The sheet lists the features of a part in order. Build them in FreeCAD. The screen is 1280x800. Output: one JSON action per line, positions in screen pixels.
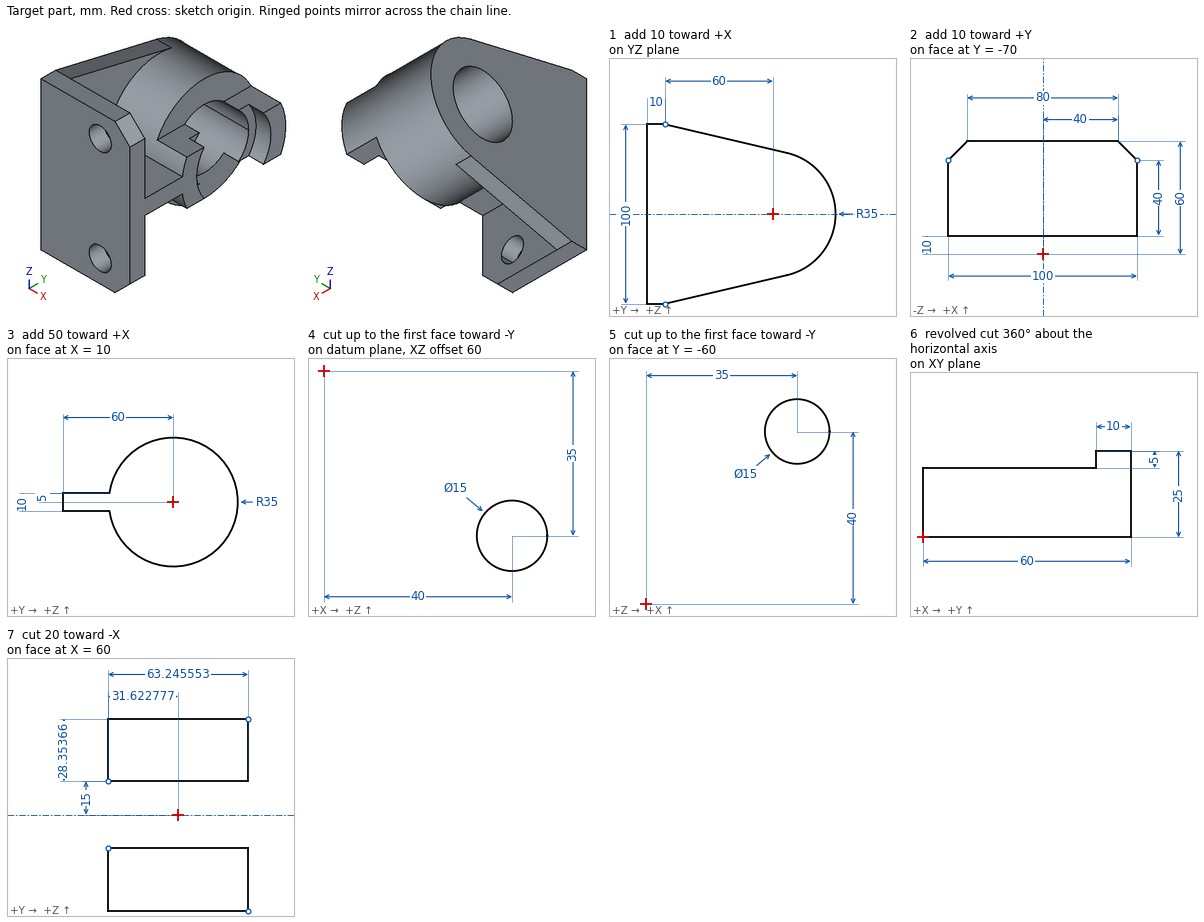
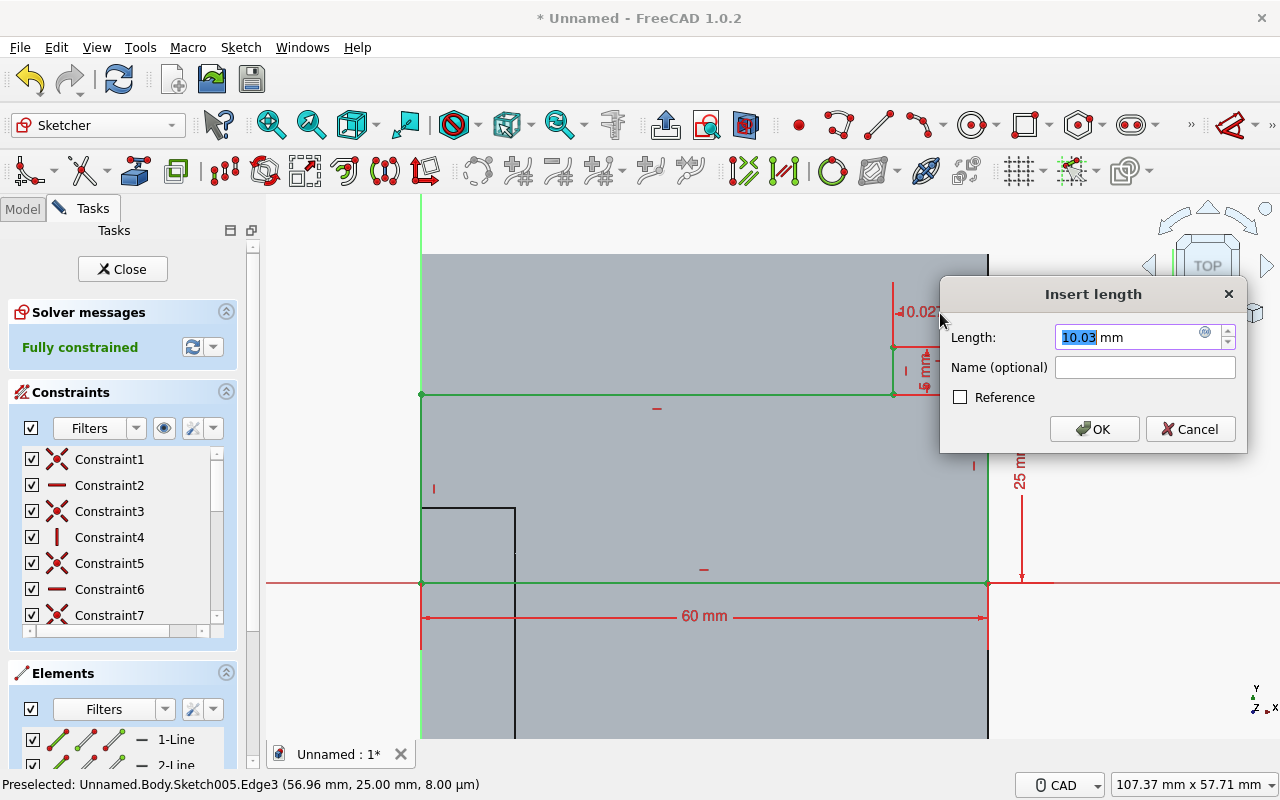
{"action": "type", "text": "10"}
{"action": "key", "text": "Return"}
{"action": "key", "text": "Escape"}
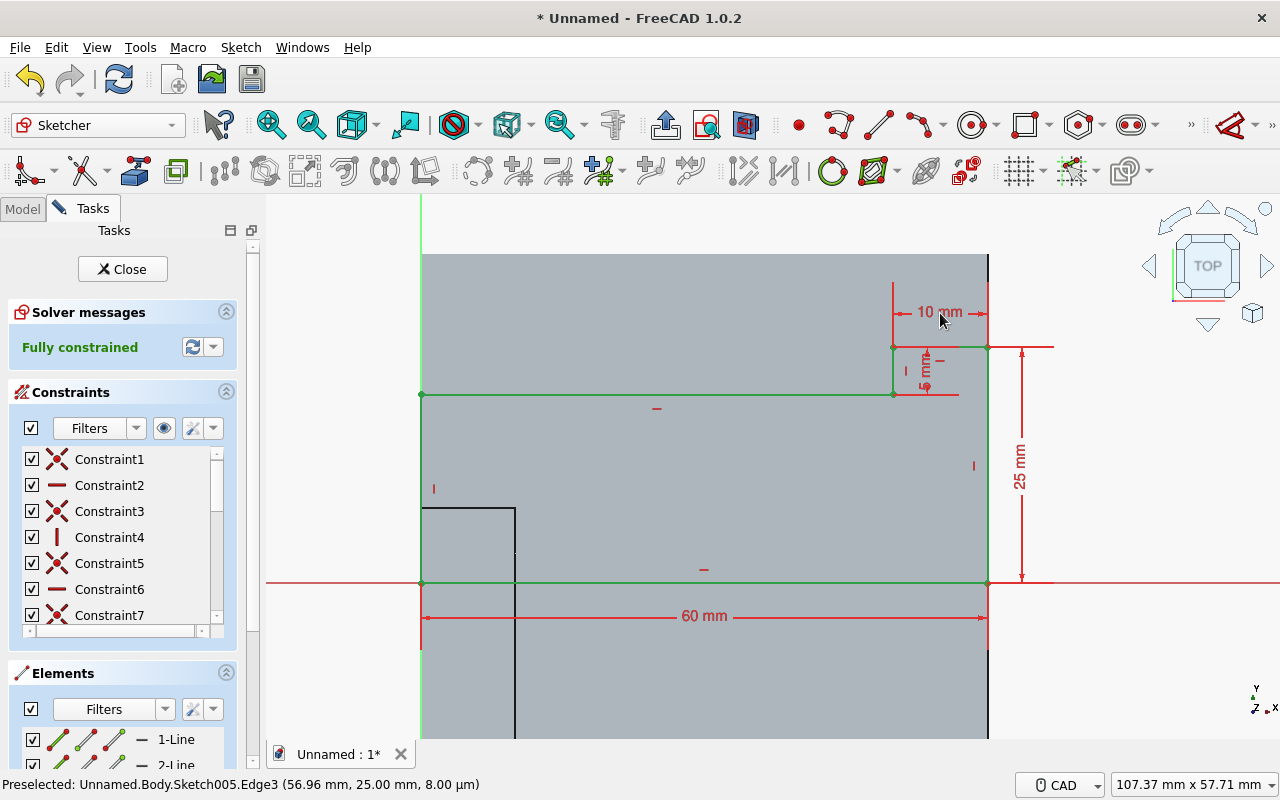
{"action": "left_click", "coordinate": [123, 269]}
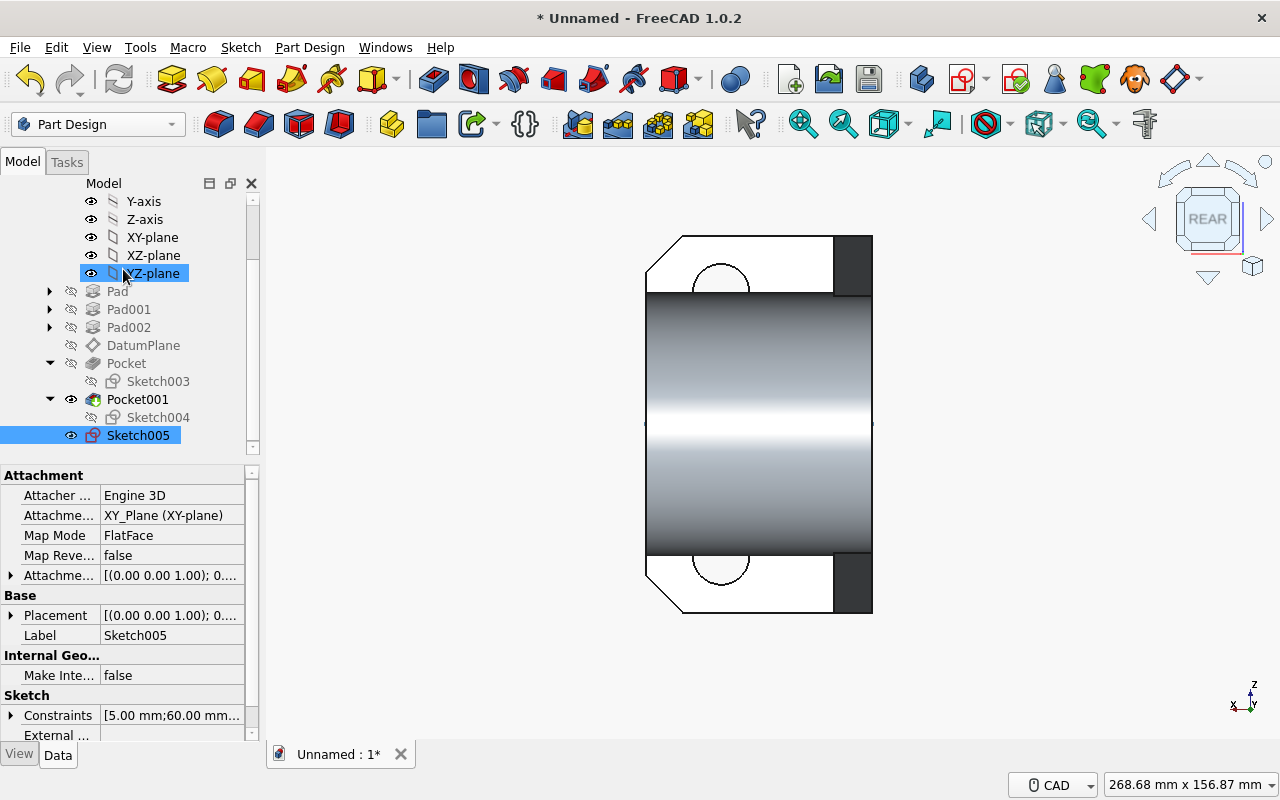
{"action": "left_click", "coordinate": [514, 80]}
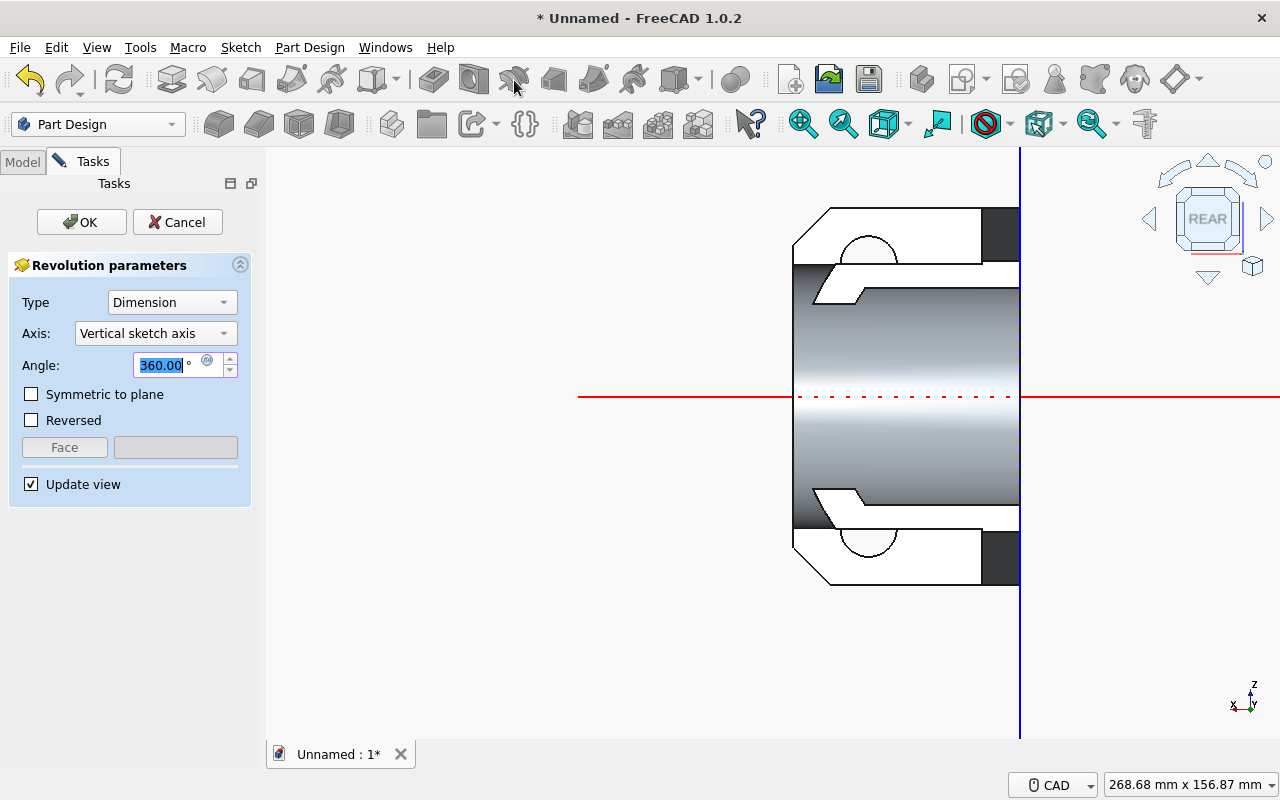
{"action": "left_click", "coordinate": [156, 334]}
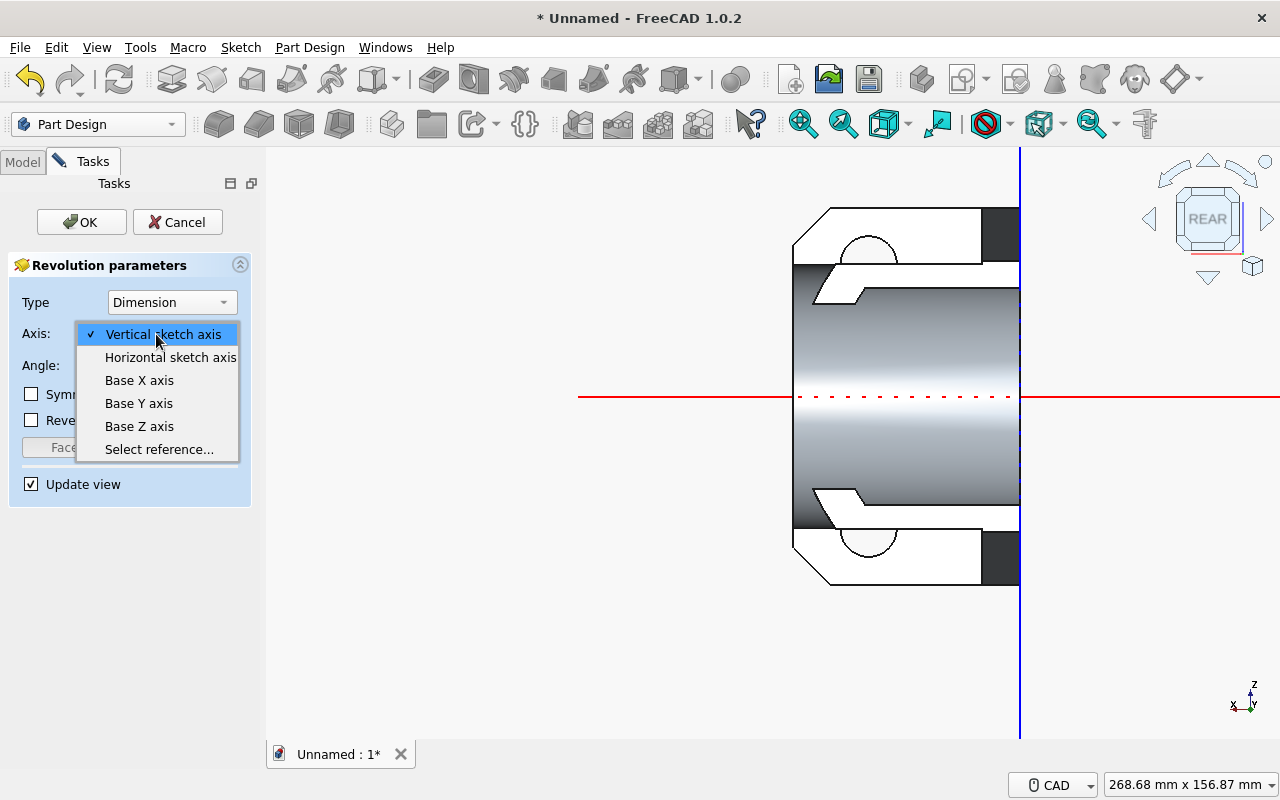
{"action": "left_click", "coordinate": [156, 358]}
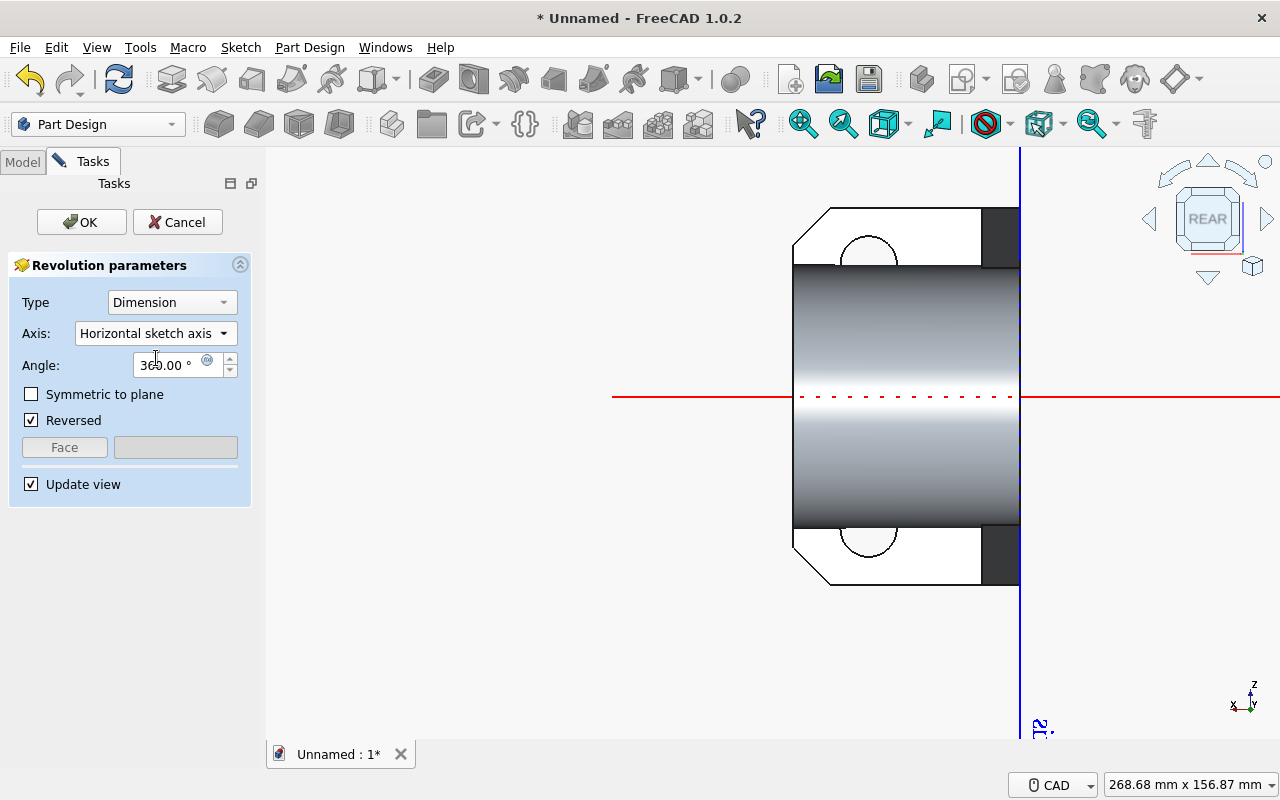
{"action": "left_click", "coordinate": [82, 222]}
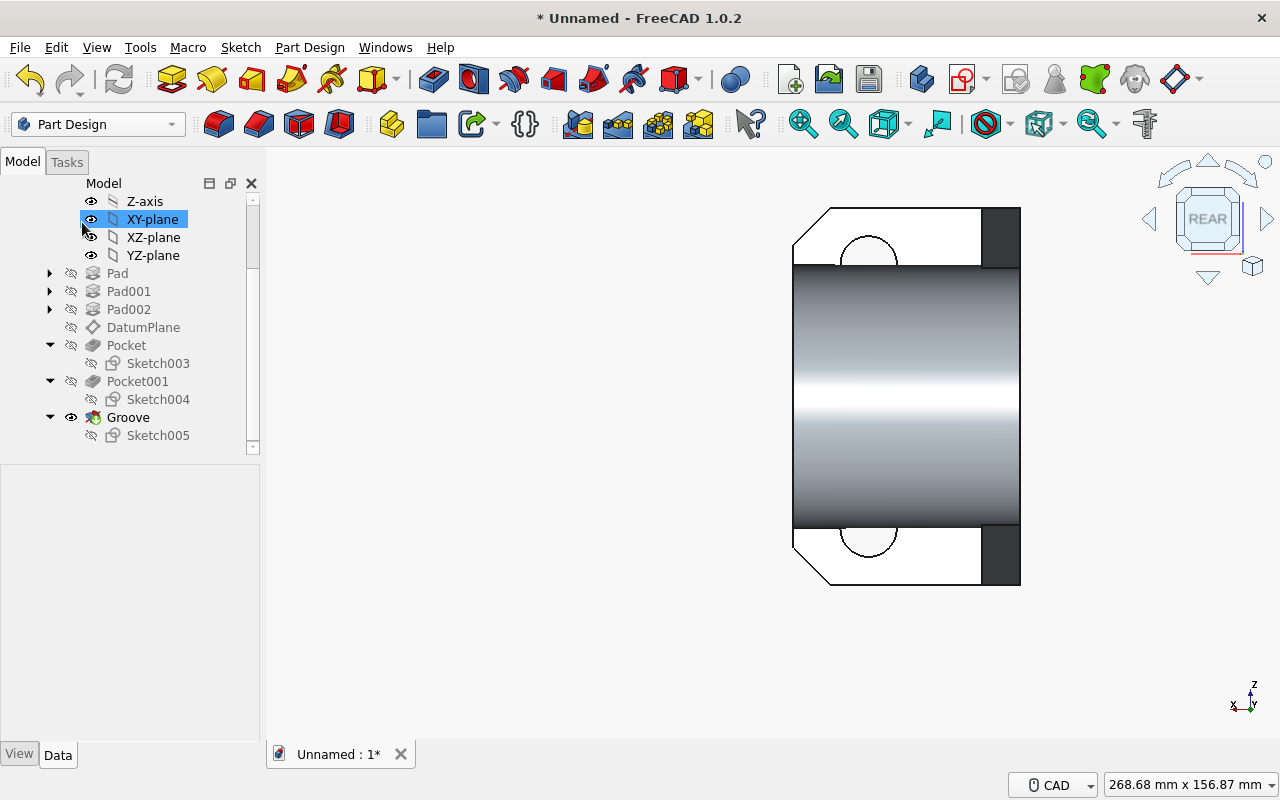
{"action": "key", "text": "0"}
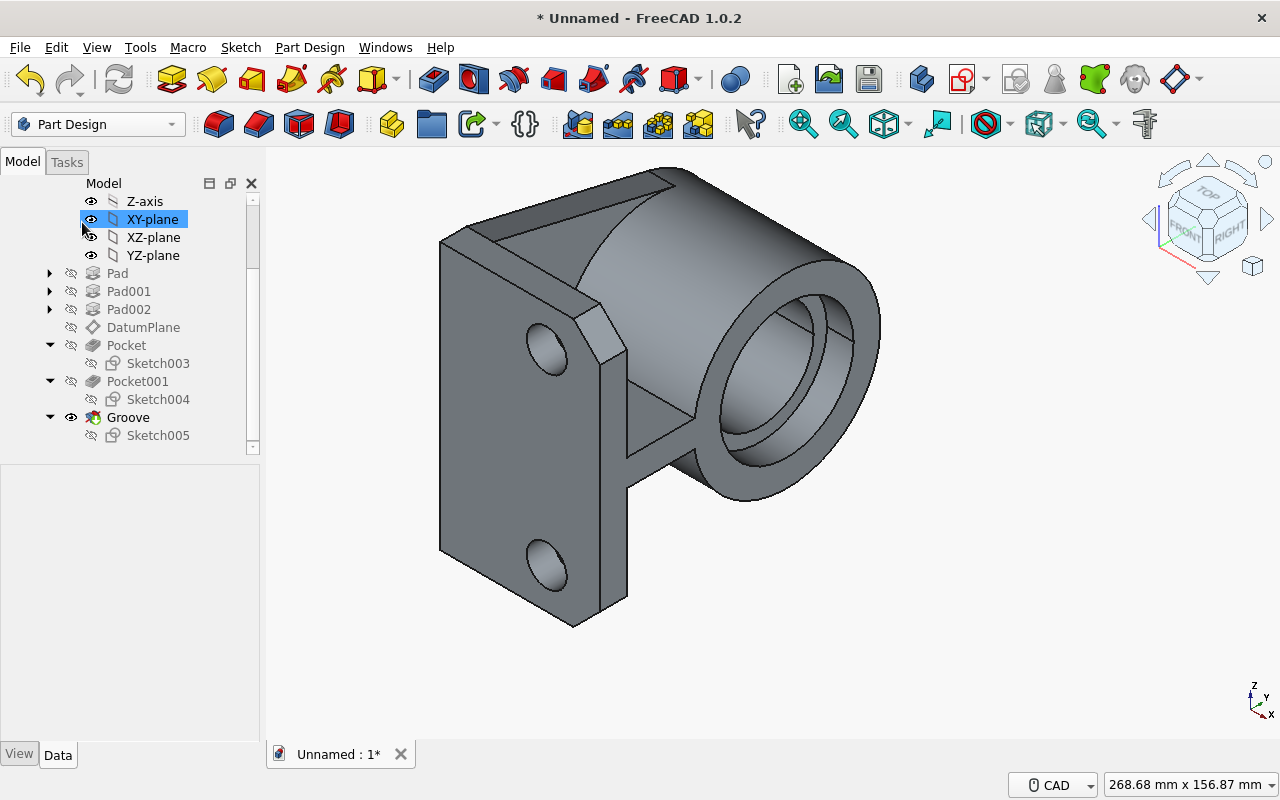
{"action": "left_click", "coordinate": [804, 124]}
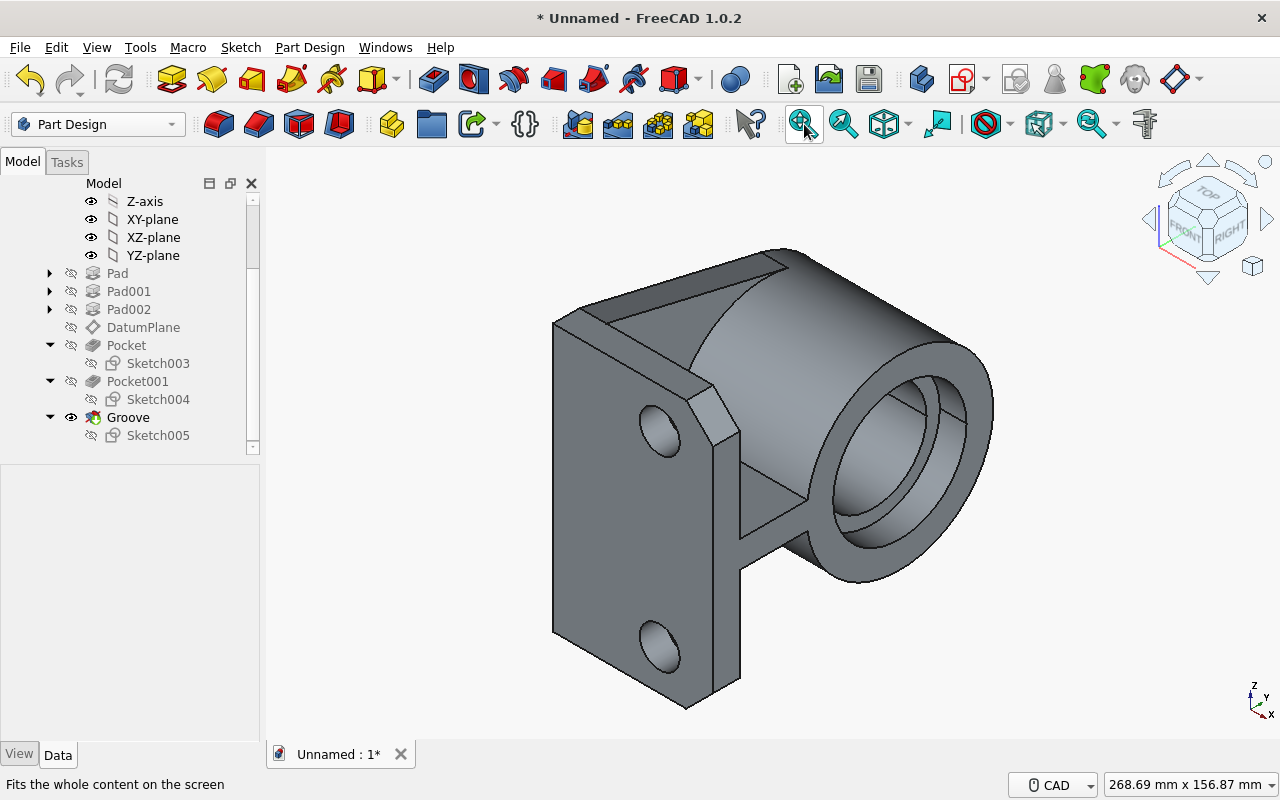
{"action": "left_click", "coordinate": [733, 557]}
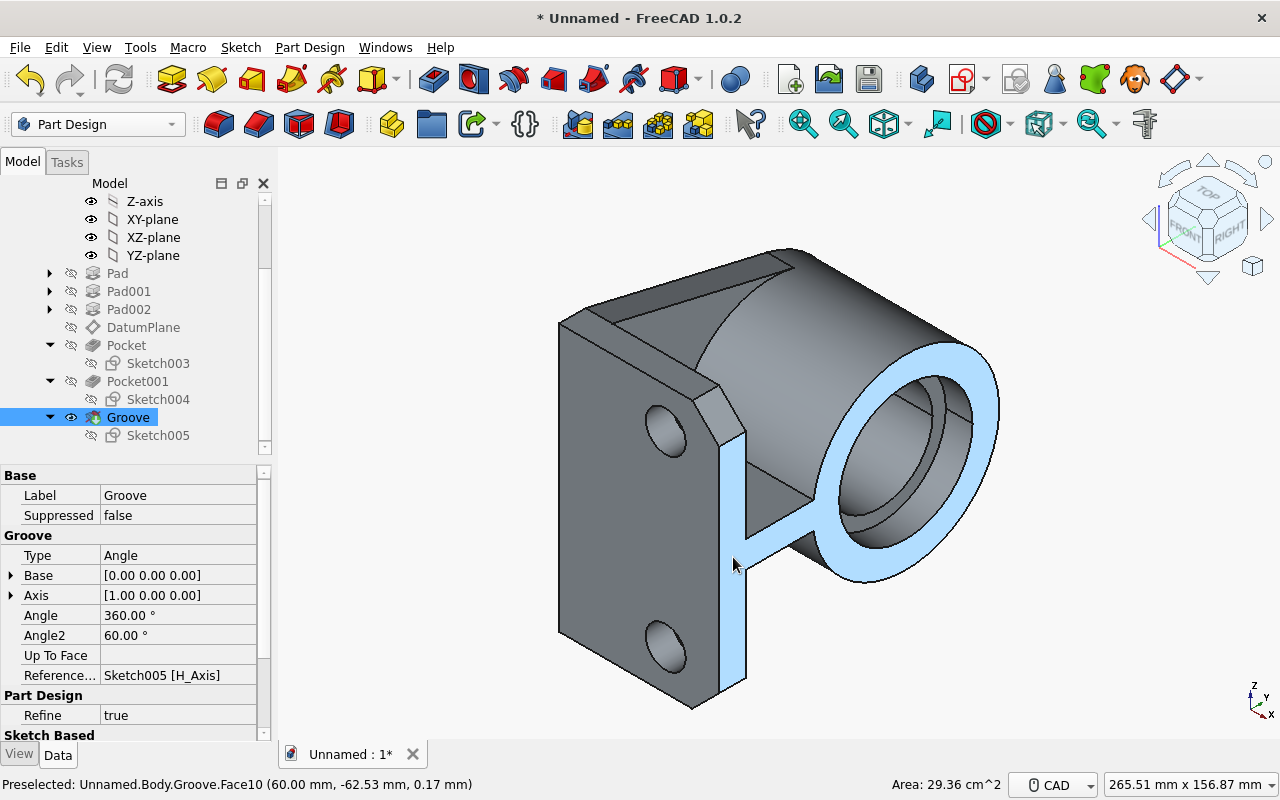
{"action": "left_click", "coordinate": [962, 80]}